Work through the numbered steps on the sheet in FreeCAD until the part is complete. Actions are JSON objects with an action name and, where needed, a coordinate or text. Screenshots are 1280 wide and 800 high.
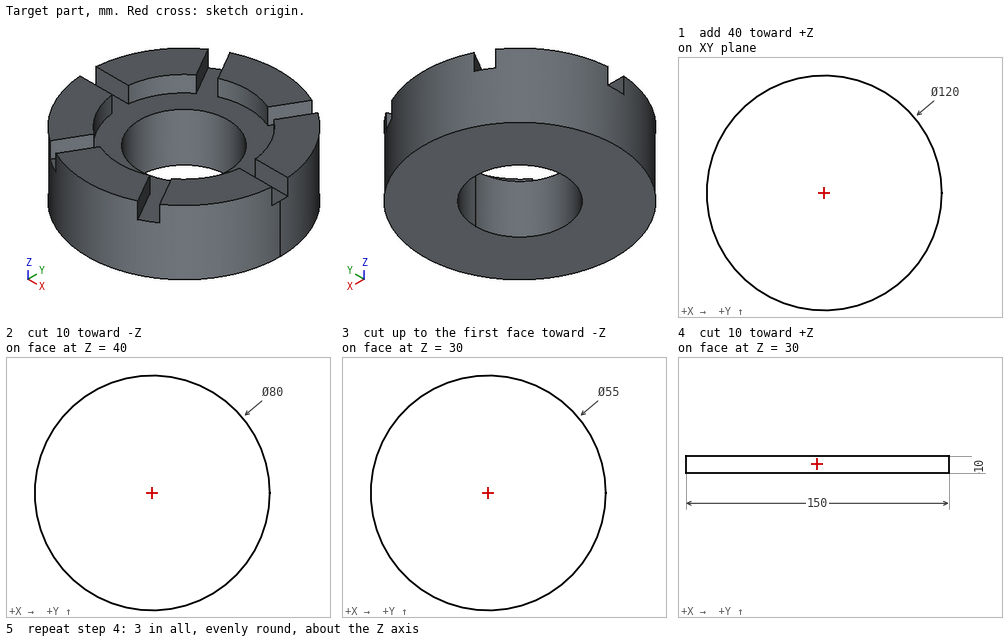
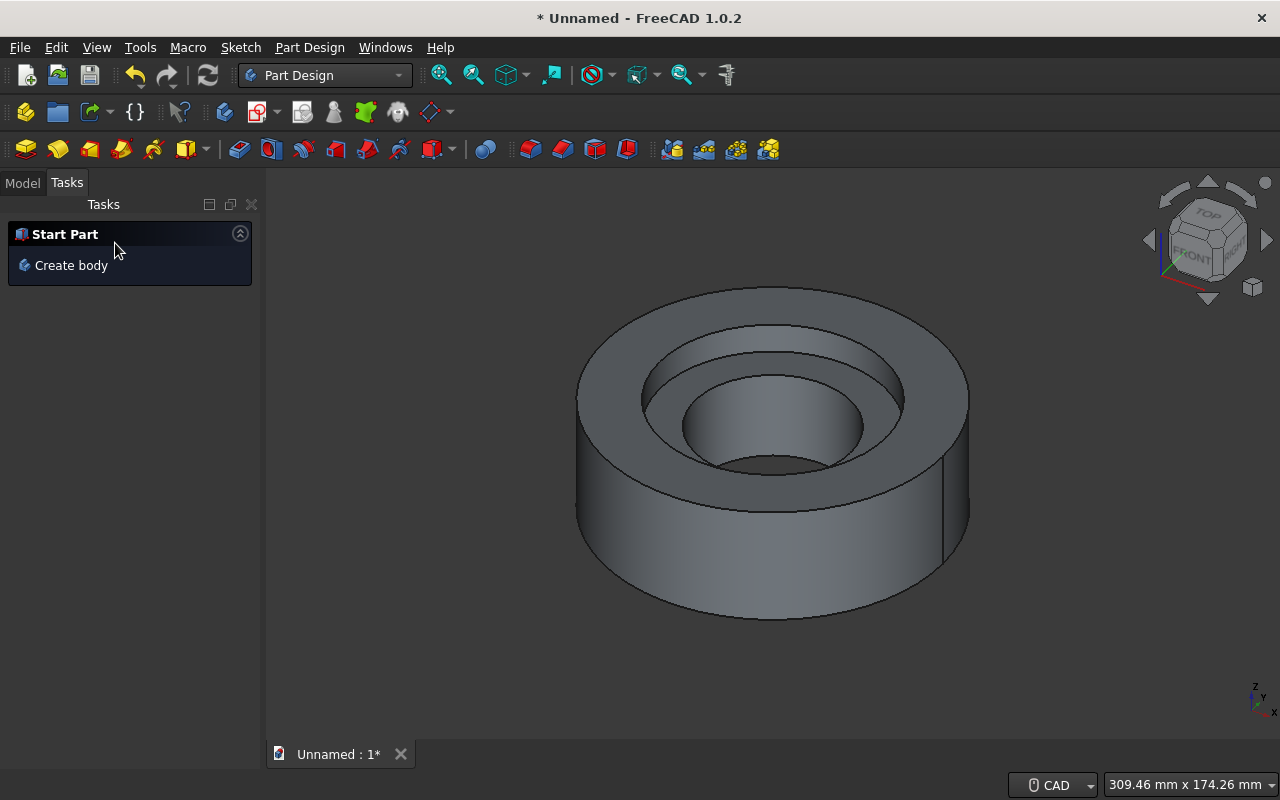
{"action": "left_click", "coordinate": [676, 393]}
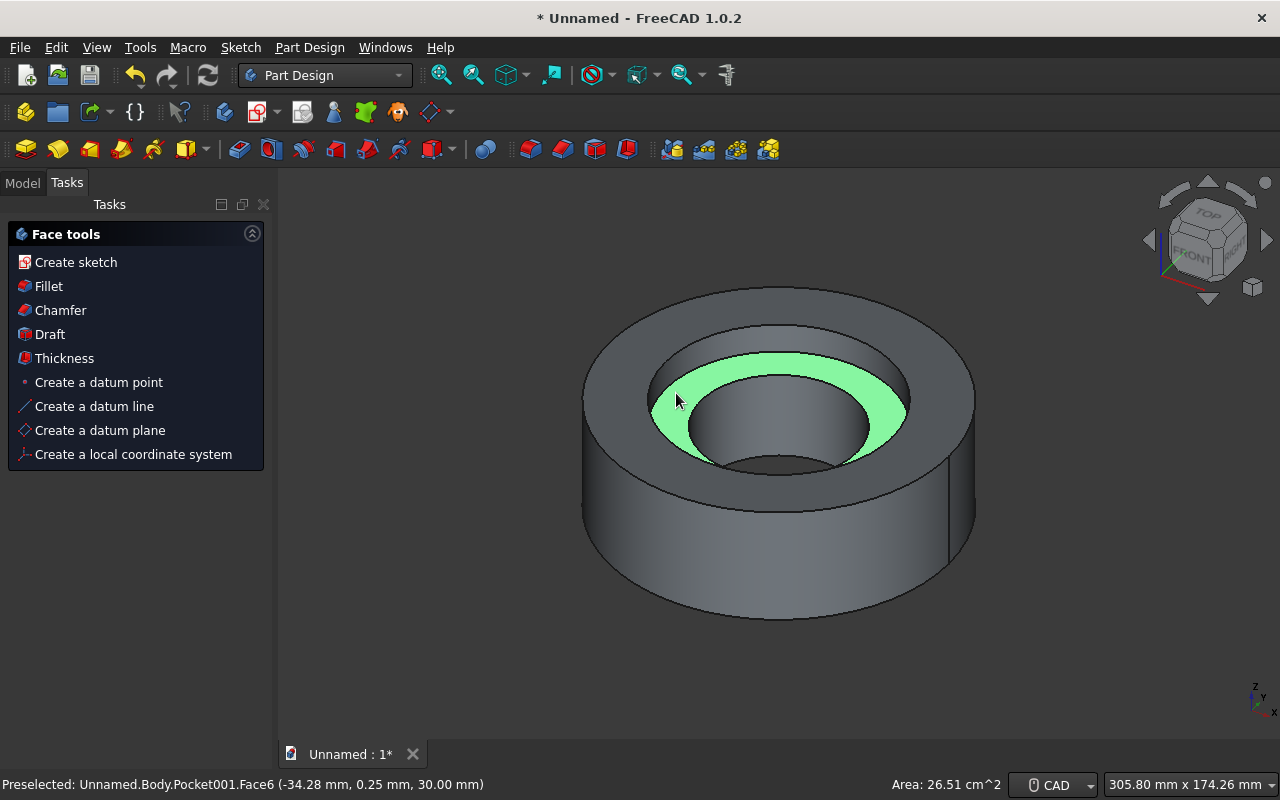
{"action": "left_click", "coordinate": [258, 112]}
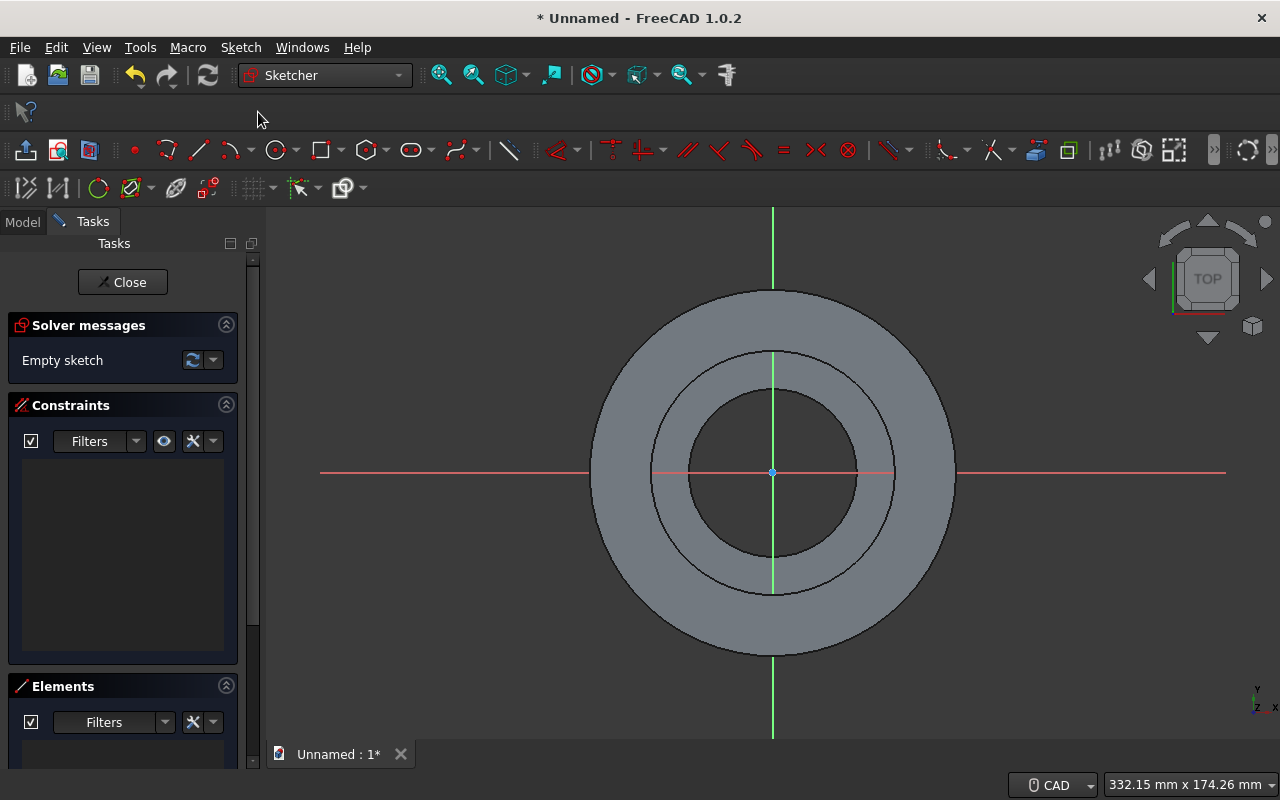
{"action": "key", "text": "g v"}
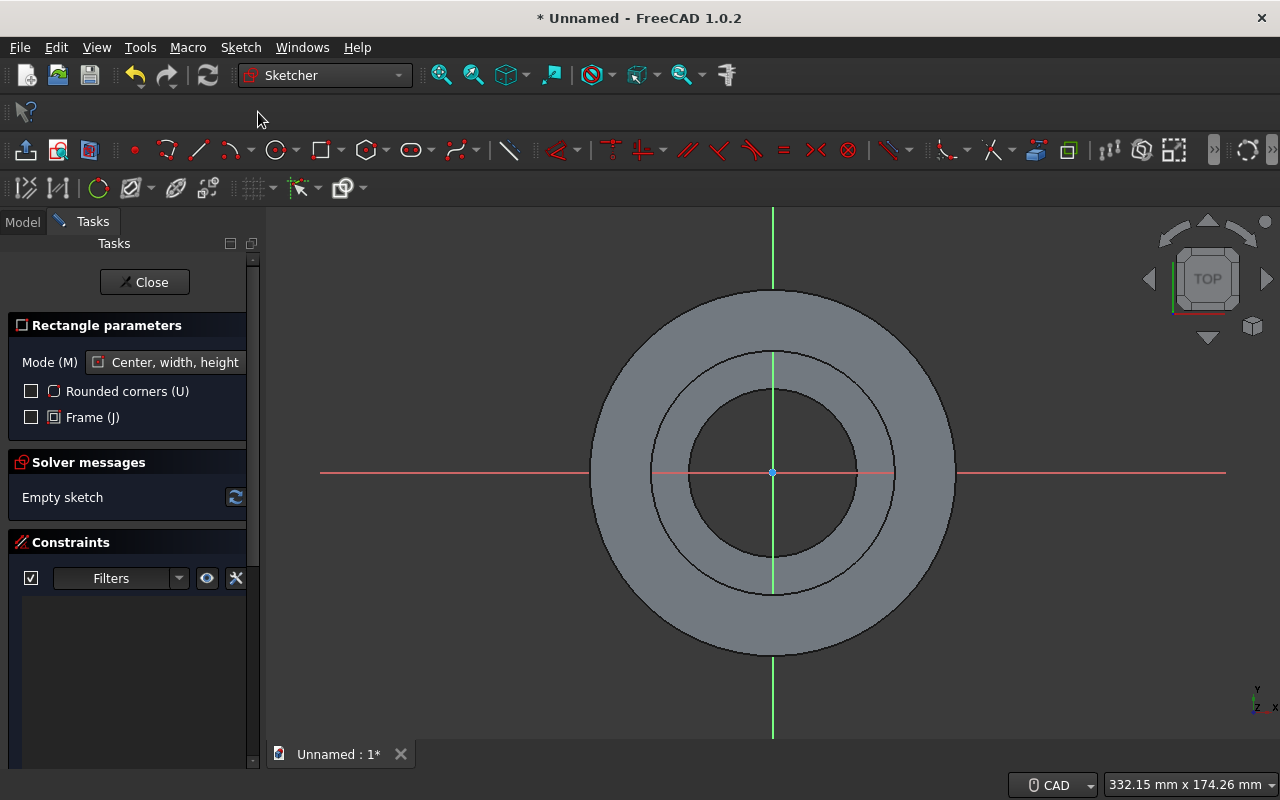
{"action": "left_click", "coordinate": [773, 473]}
{"action": "left_click", "coordinate": [1002, 458]}
{"action": "key", "text": "Escape"}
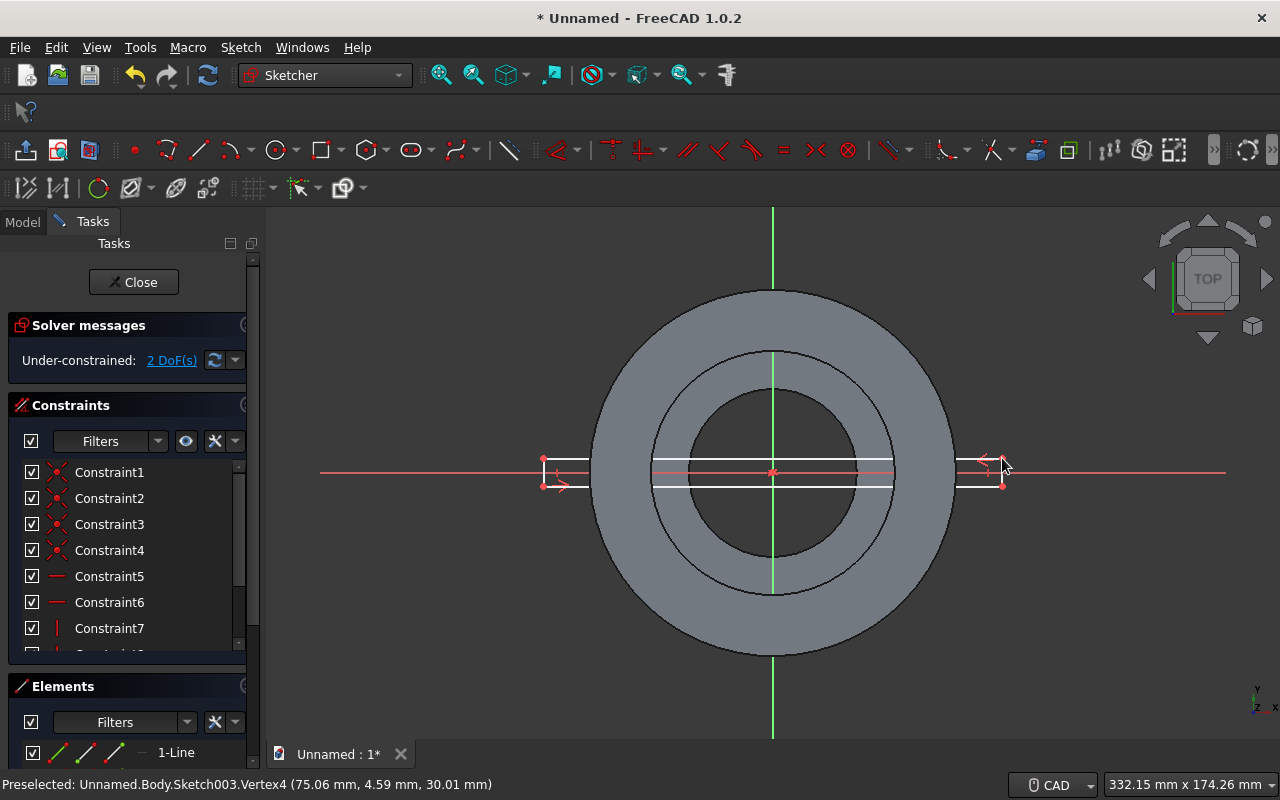
{"action": "key", "text": "d"}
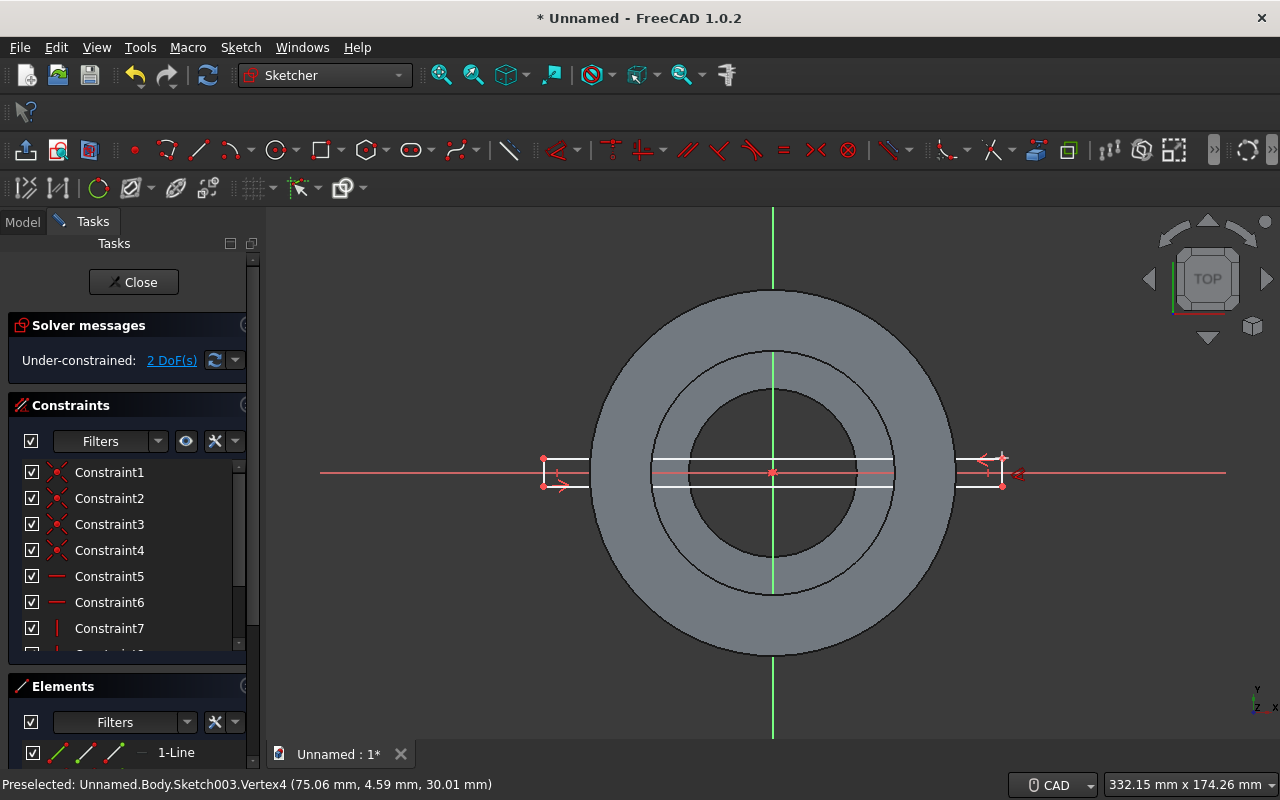
{"action": "scroll", "coordinate": [1002, 476], "scroll_direction": "up", "scroll_amount": 2}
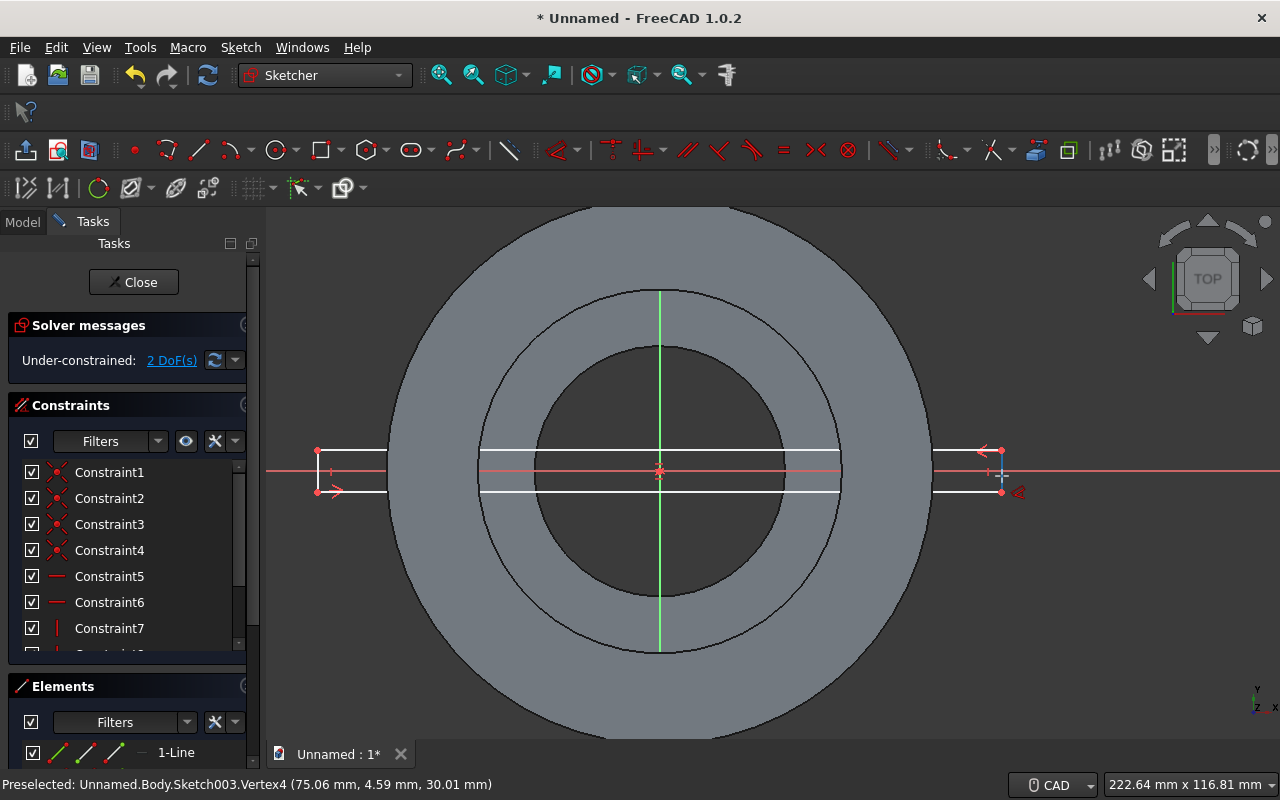
{"action": "left_click", "coordinate": [1002, 475]}
{"action": "left_click", "coordinate": [1036, 457]}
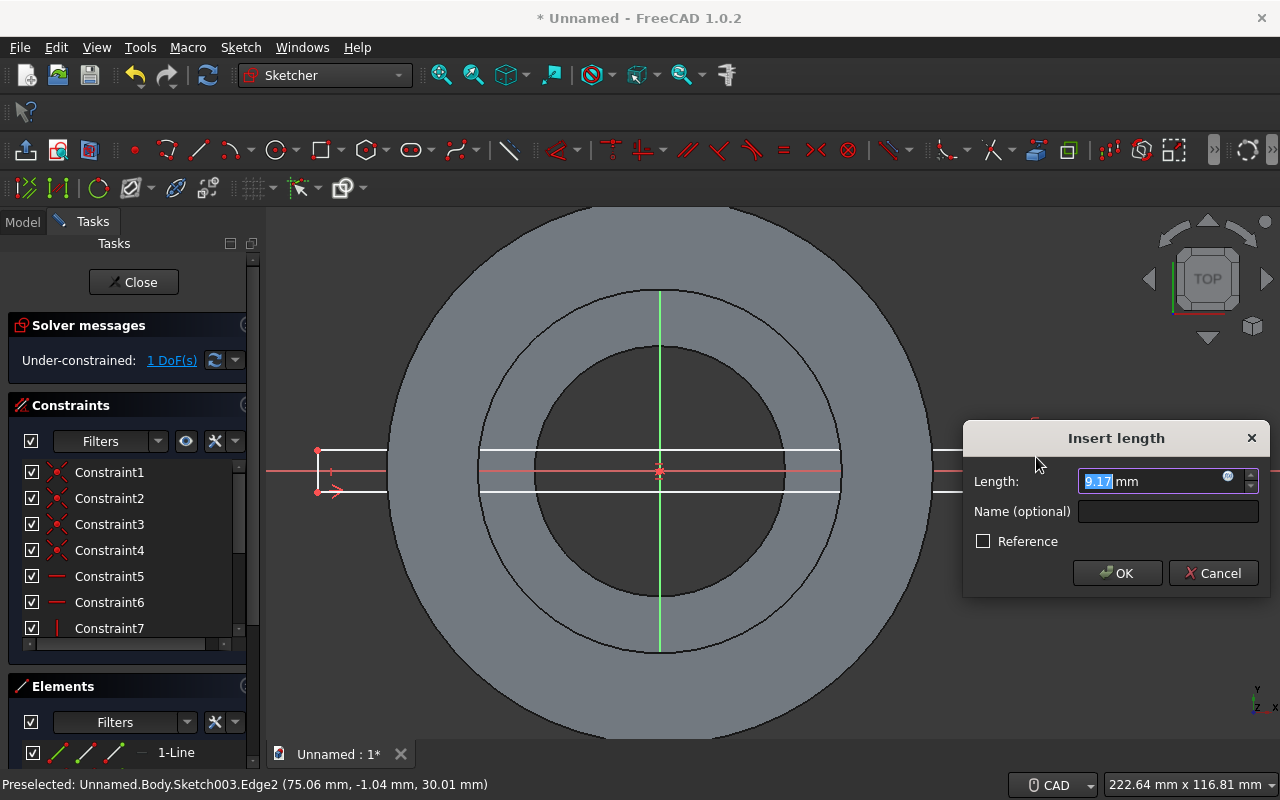
{"action": "type", "text": "10"}
{"action": "key", "text": "Return"}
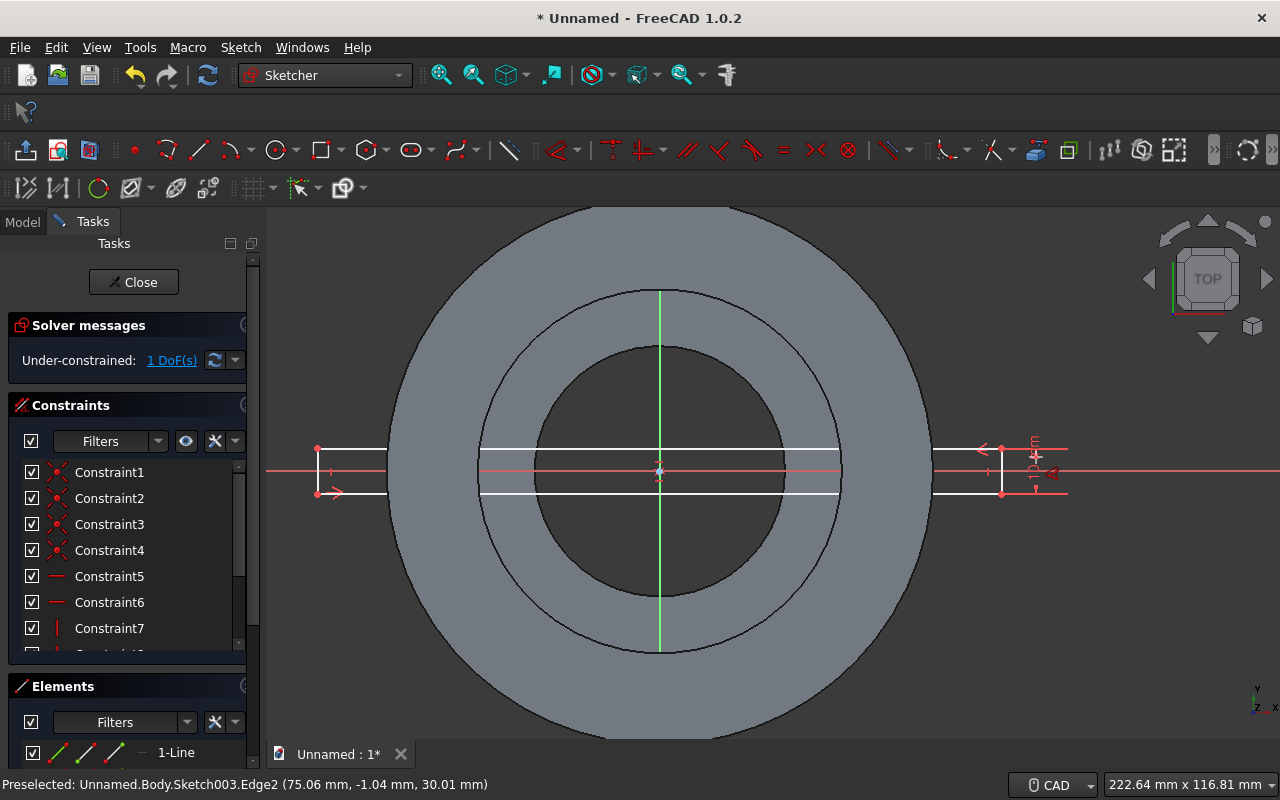
{"action": "left_click", "coordinate": [523, 494]}
{"action": "left_click", "coordinate": [503, 528]}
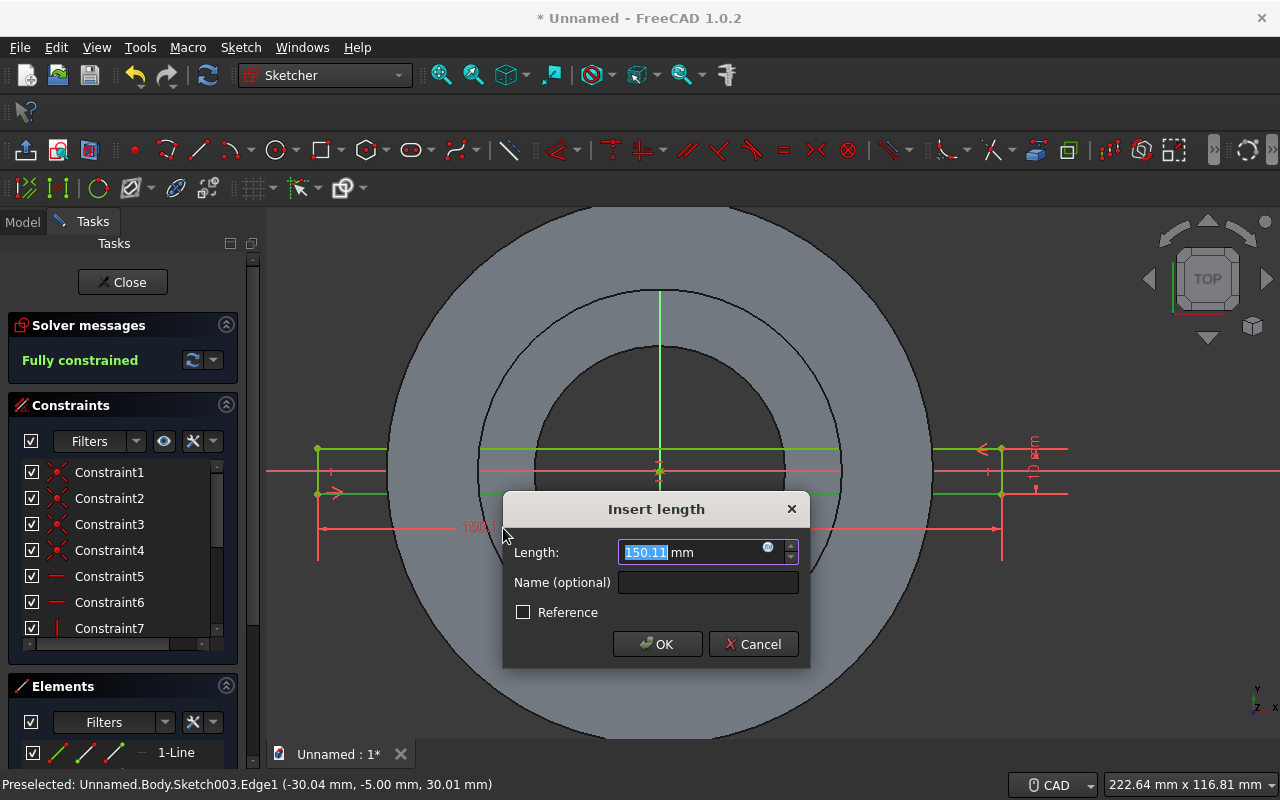
{"action": "type", "text": "150"}
{"action": "key", "text": "Return"}
{"action": "key", "text": "Escape"}